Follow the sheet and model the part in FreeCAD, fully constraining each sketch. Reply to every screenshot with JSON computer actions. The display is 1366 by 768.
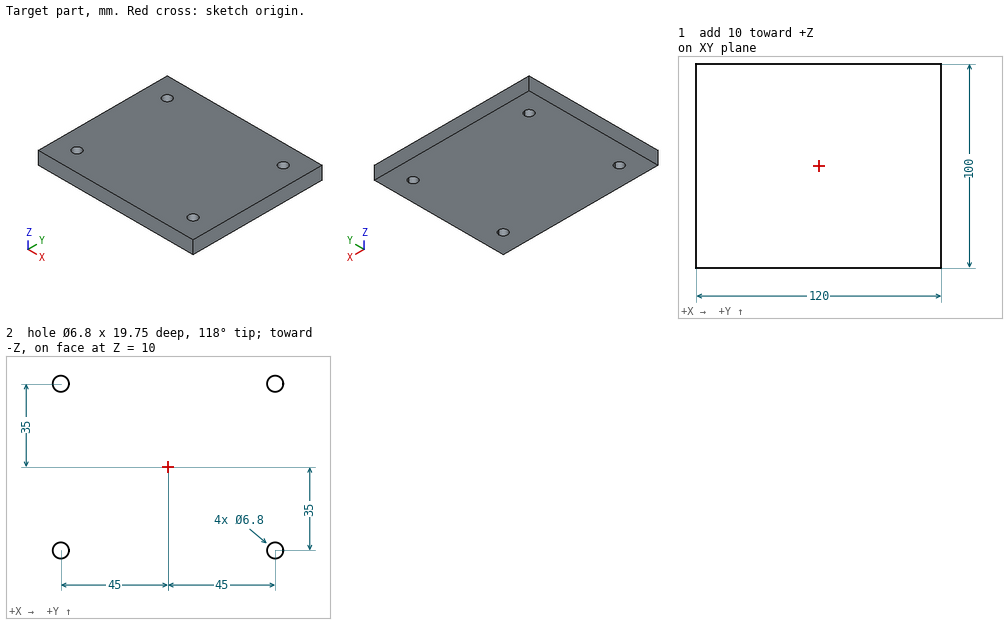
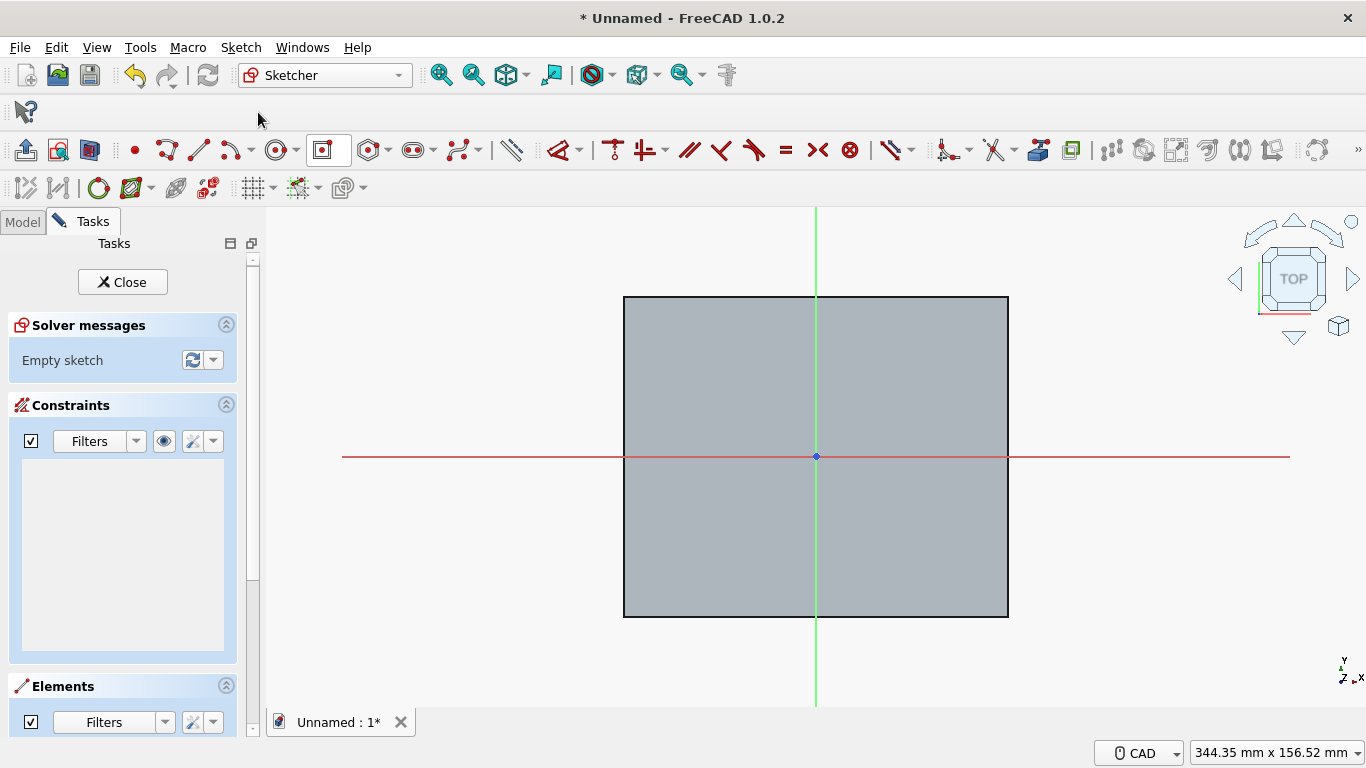
{"action": "left_click", "coordinate": [276, 150]}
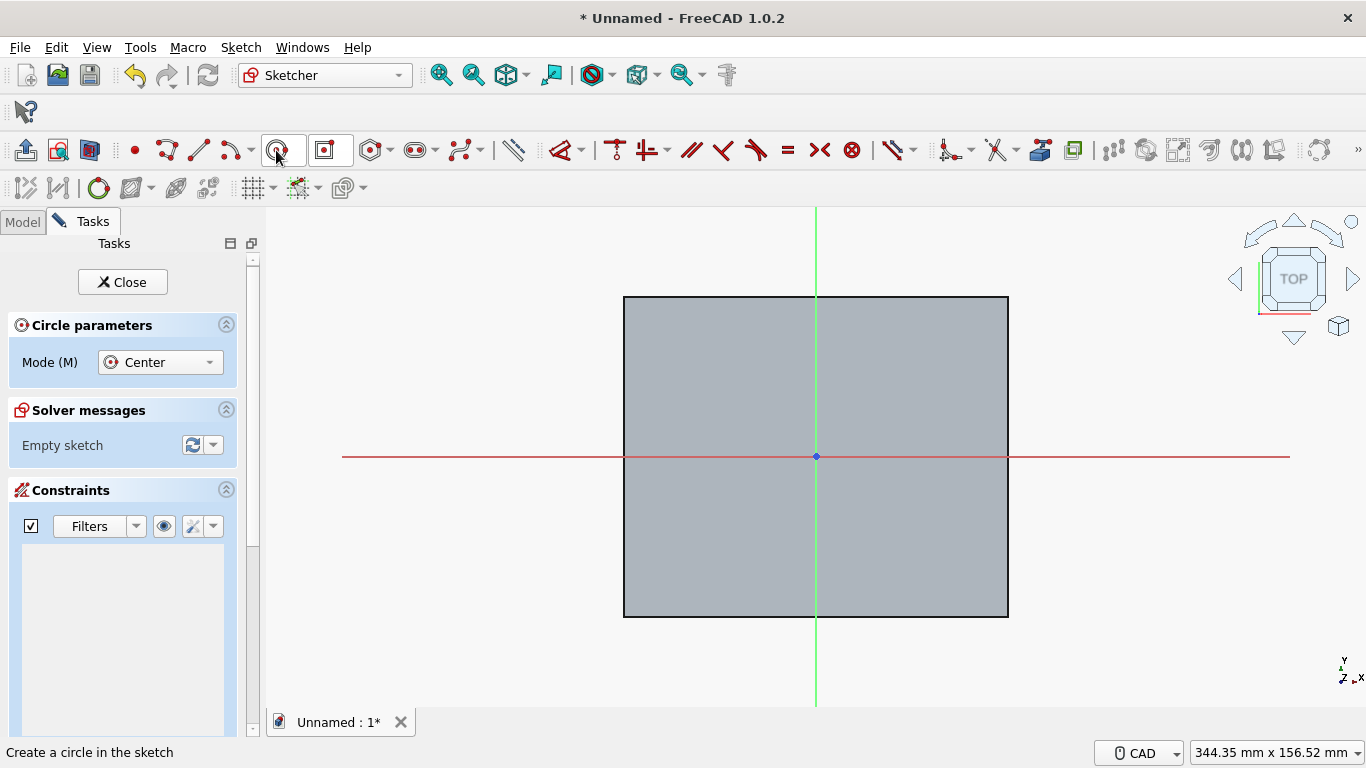
{"action": "scroll", "coordinate": [960, 569], "scroll_direction": "up", "scroll_amount": 4}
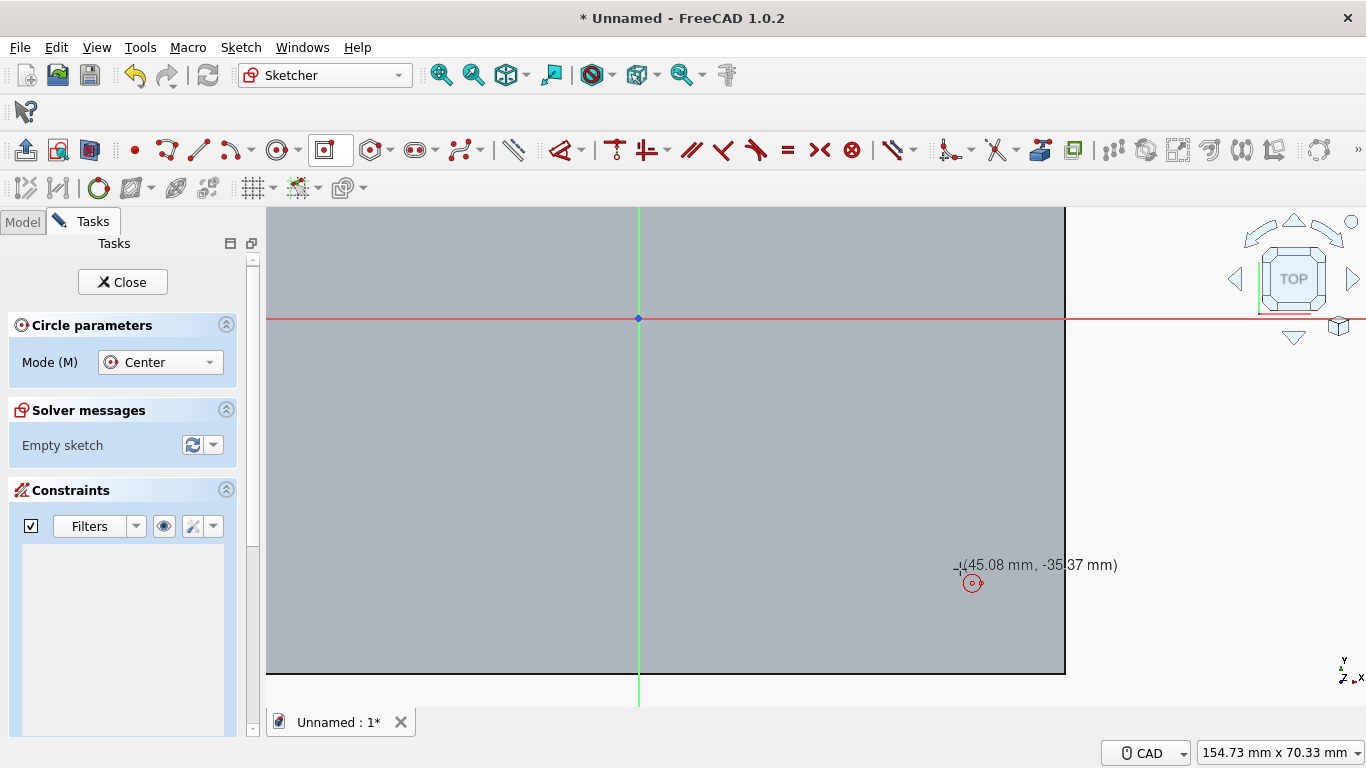
{"action": "left_click", "coordinate": [959, 568]}
{"action": "left_click", "coordinate": [976, 551]}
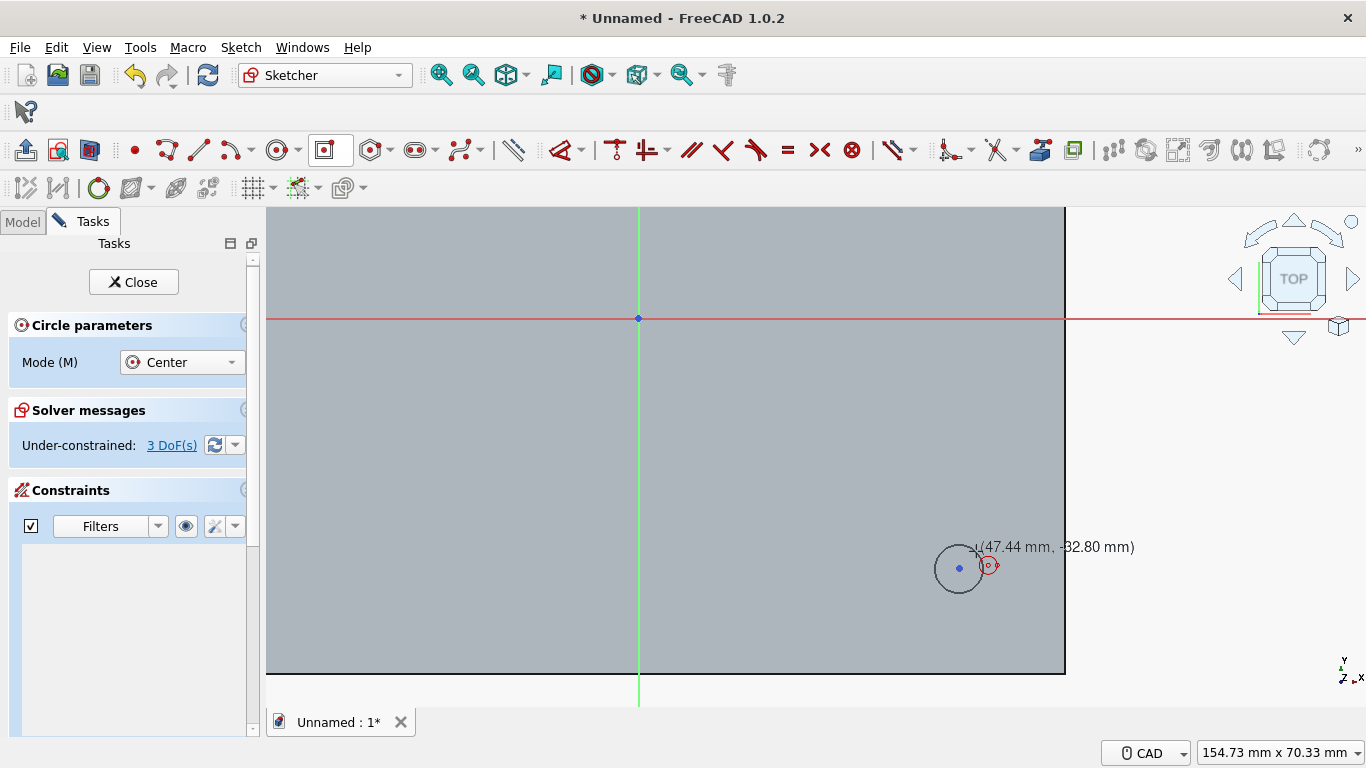
{"action": "left_click", "coordinate": [319, 568]}
{"action": "left_click", "coordinate": [336, 551]}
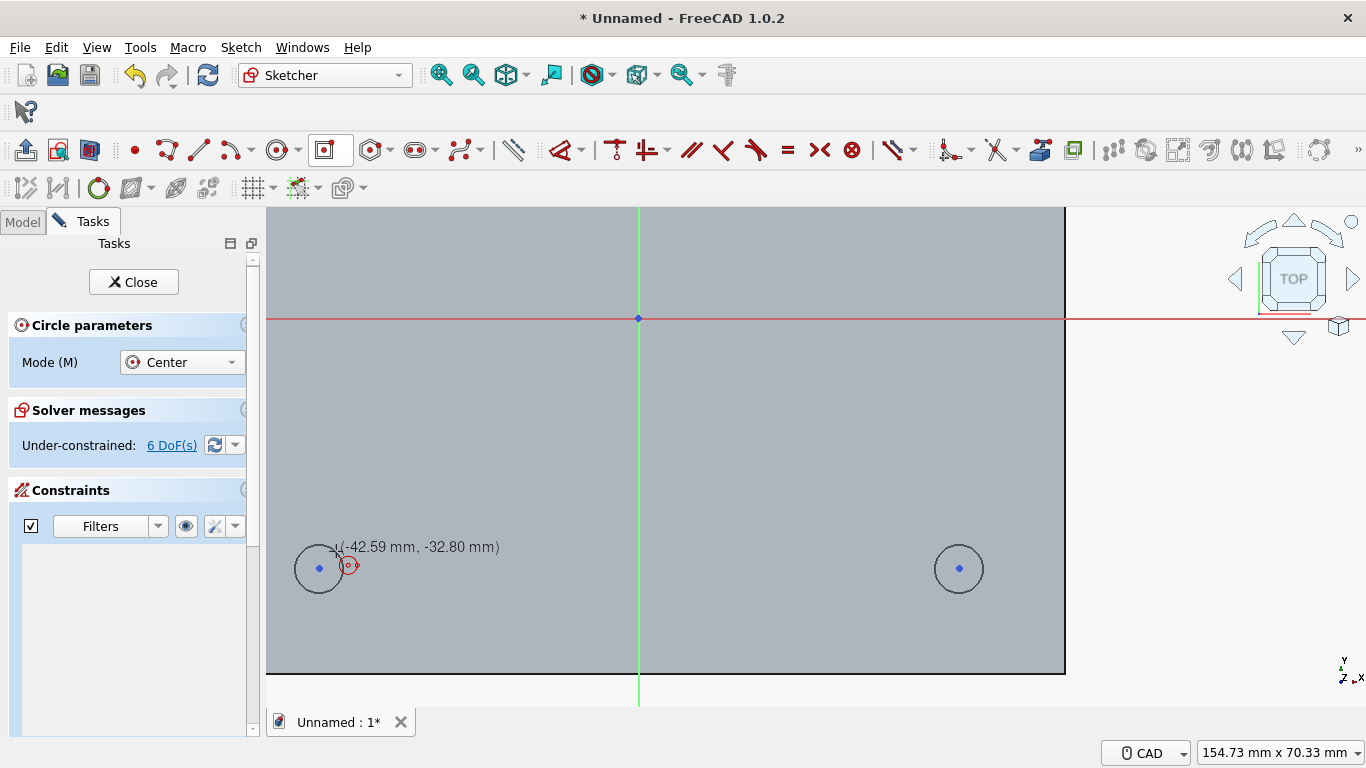
{"action": "scroll", "coordinate": [880, 625], "scroll_direction": "down", "scroll_amount": 3}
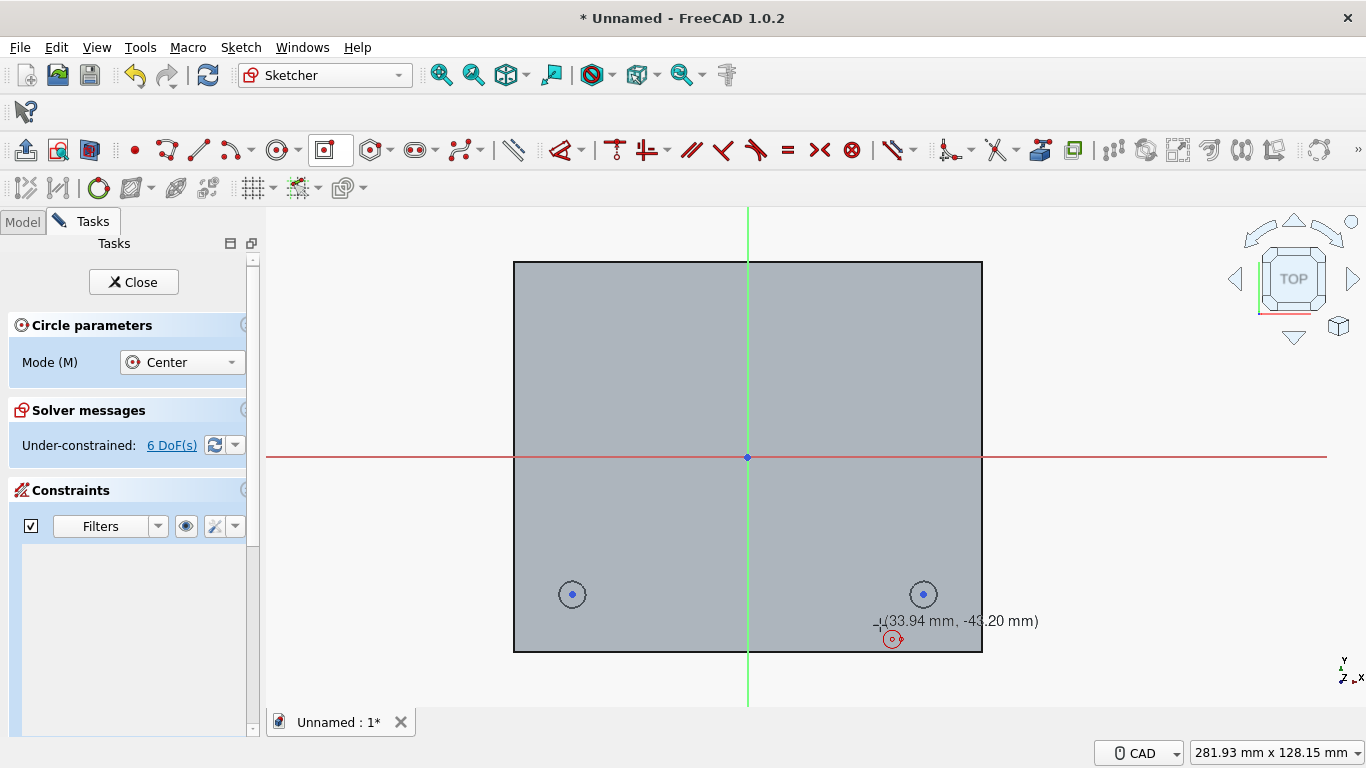
{"action": "scroll", "coordinate": [572, 321], "scroll_direction": "up", "scroll_amount": 3}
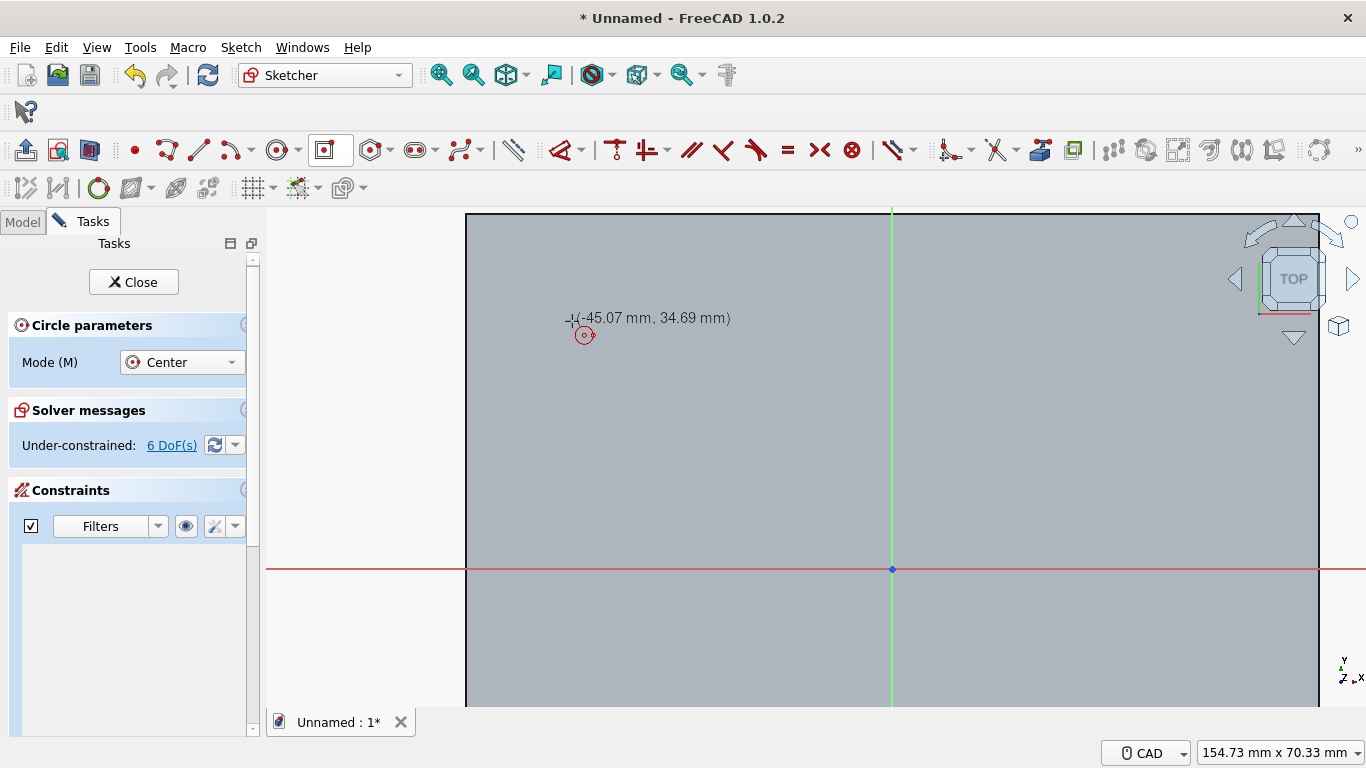
{"action": "left_click", "coordinate": [572, 320]}
{"action": "left_click", "coordinate": [589, 303]}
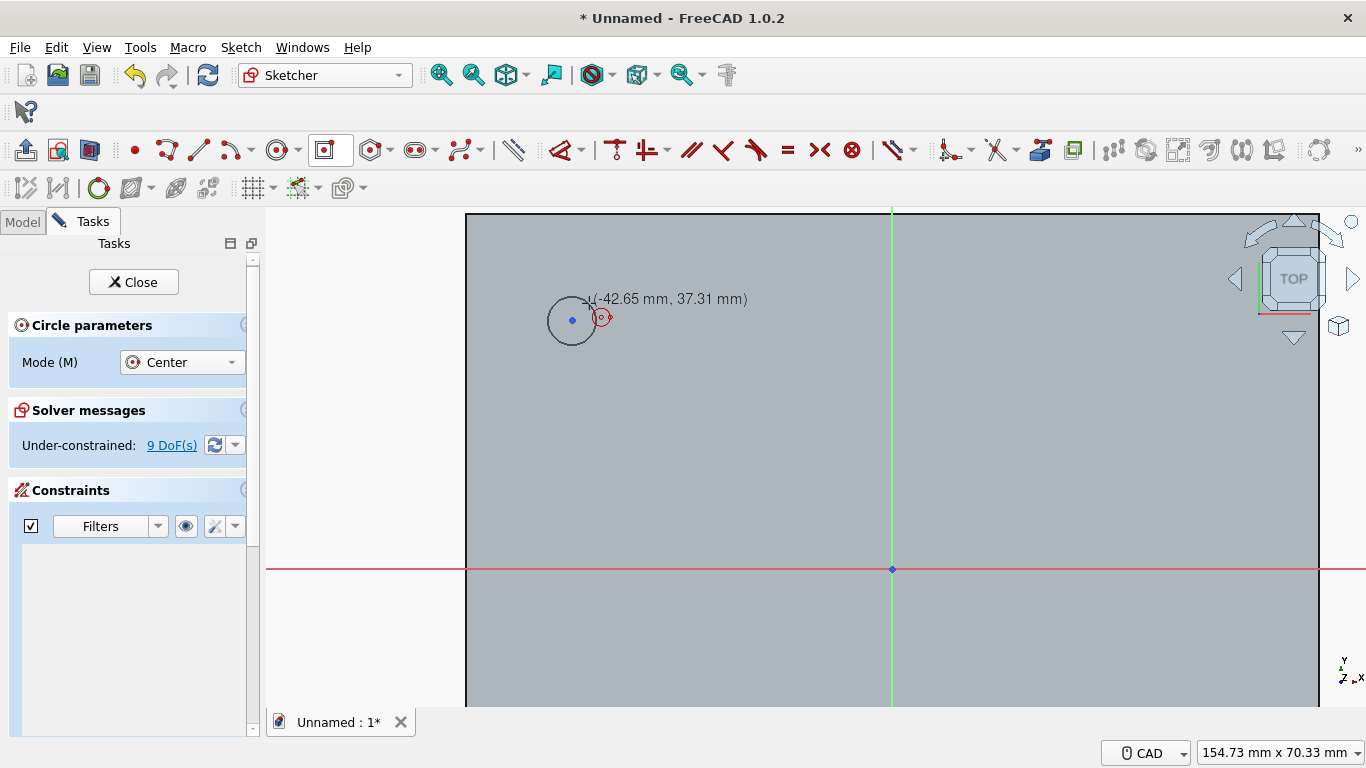
{"action": "scroll", "coordinate": [572, 320], "scroll_direction": "down", "scroll_amount": 3}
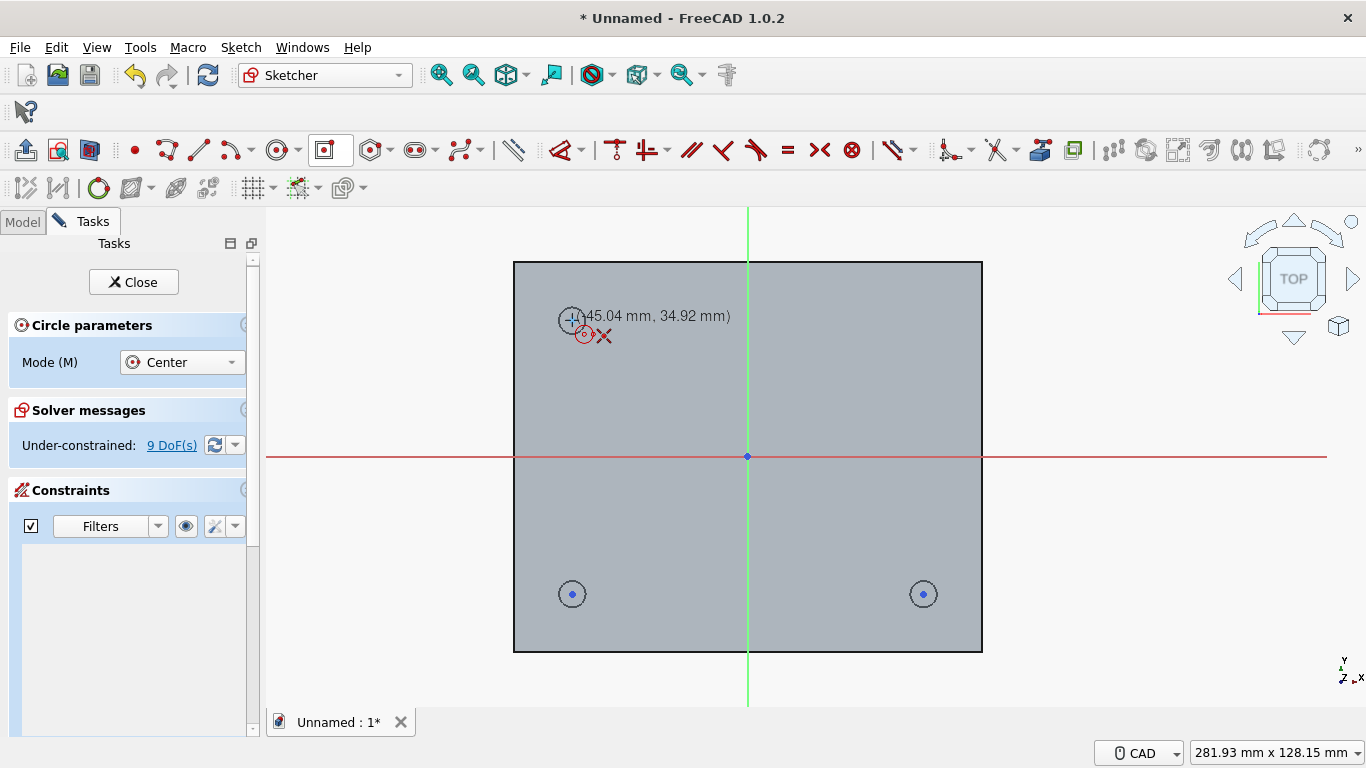
{"action": "scroll", "coordinate": [923, 320], "scroll_direction": "up", "scroll_amount": 3}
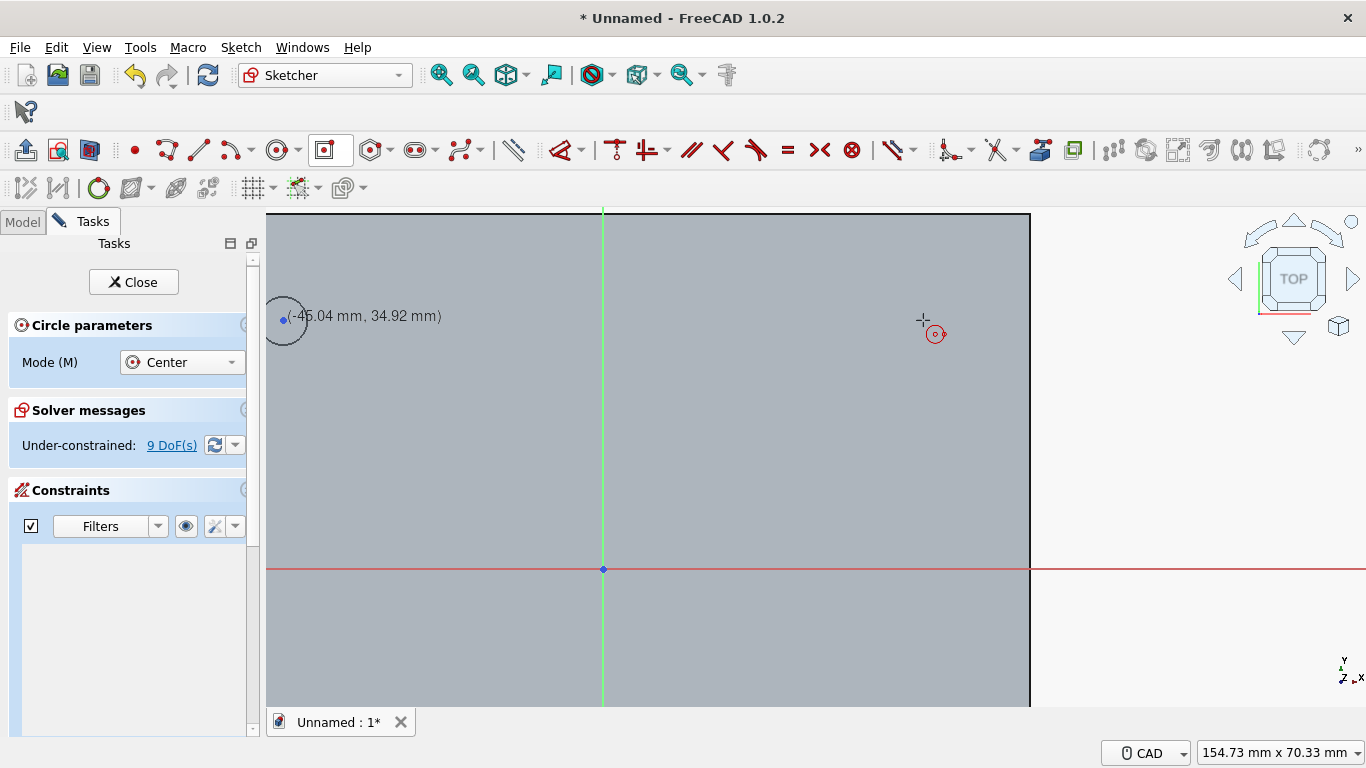
{"action": "left_click", "coordinate": [923, 320]}
{"action": "left_click", "coordinate": [940, 303]}
{"action": "key", "text": "Escape"}